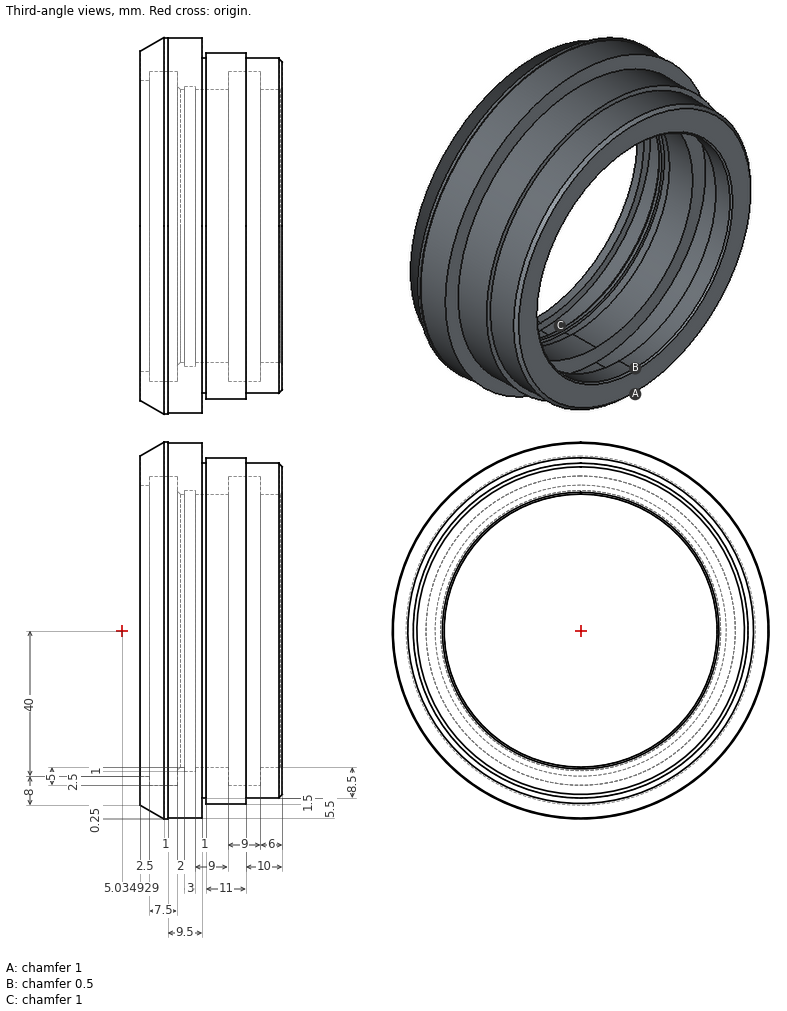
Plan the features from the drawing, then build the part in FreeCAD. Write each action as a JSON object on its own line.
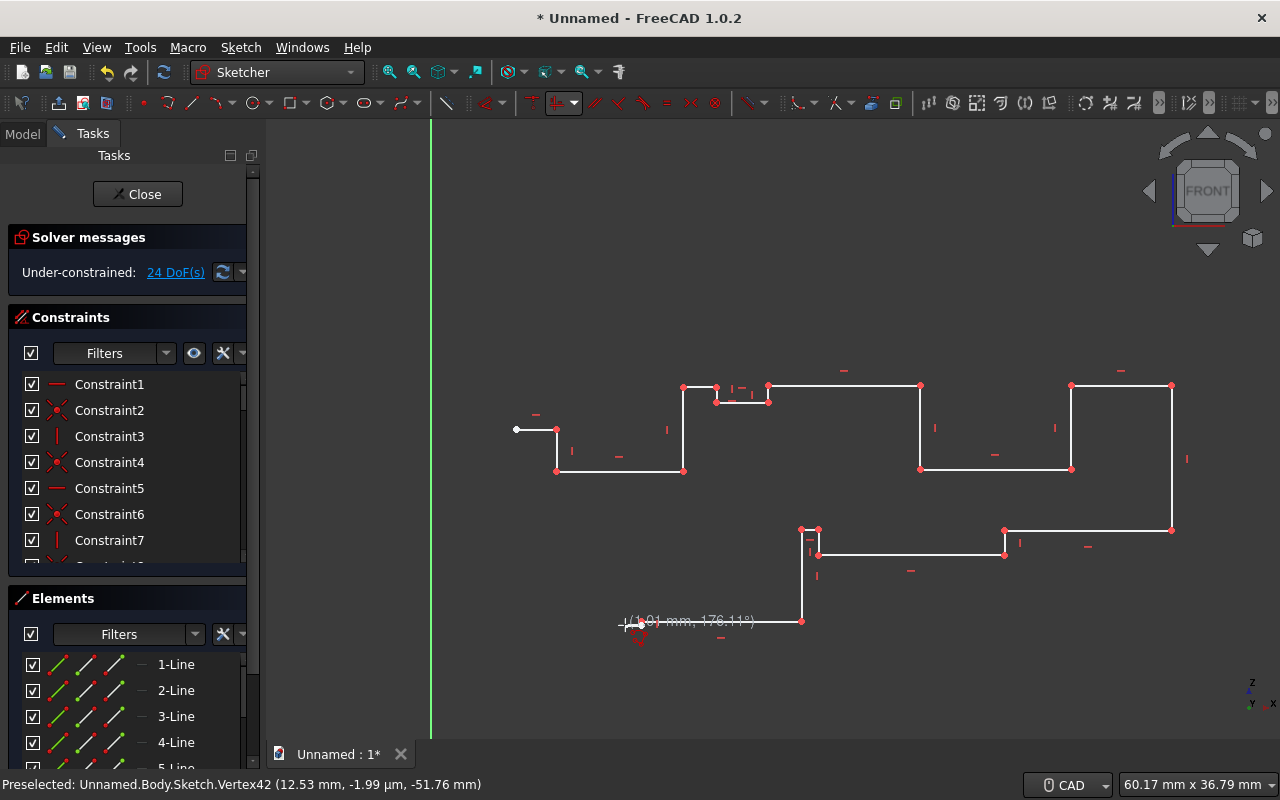
{"action": "left_click", "coordinate": [625, 625]}
{"action": "left_click", "coordinate": [515, 562]}
{"action": "left_click", "coordinate": [516, 430]}
{"action": "key", "text": "Escape"}
{"action": "key", "text": "Escape"}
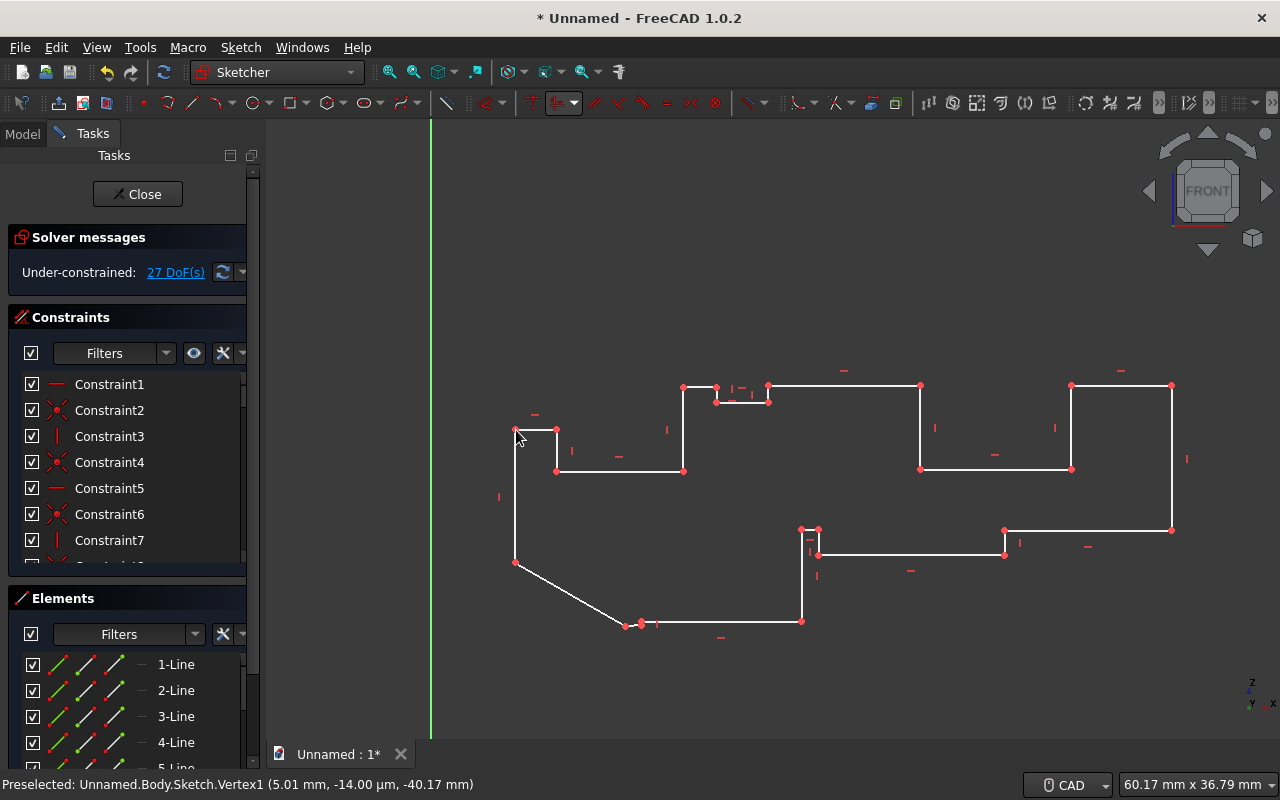
{"action": "scroll", "coordinate": [633, 626], "scroll_direction": "up", "scroll_amount": 3}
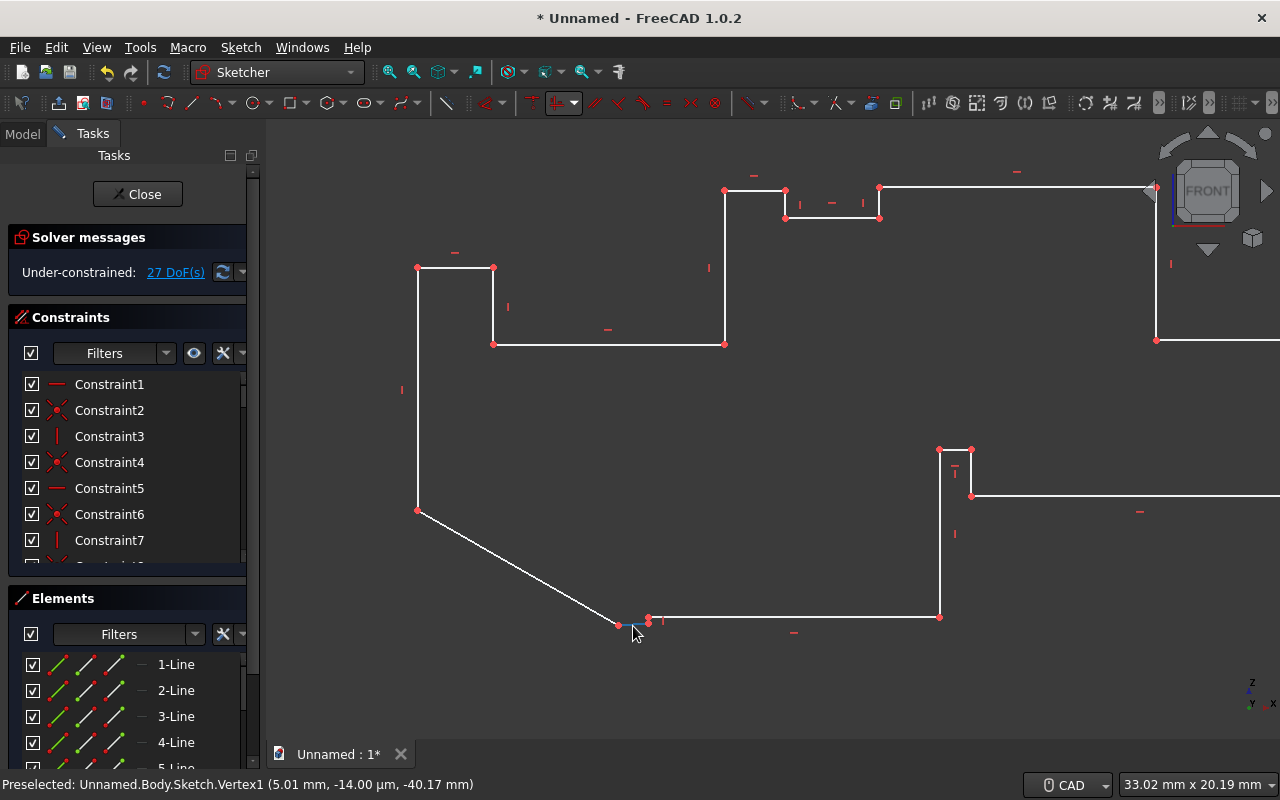
{"action": "left_click", "coordinate": [633, 624]}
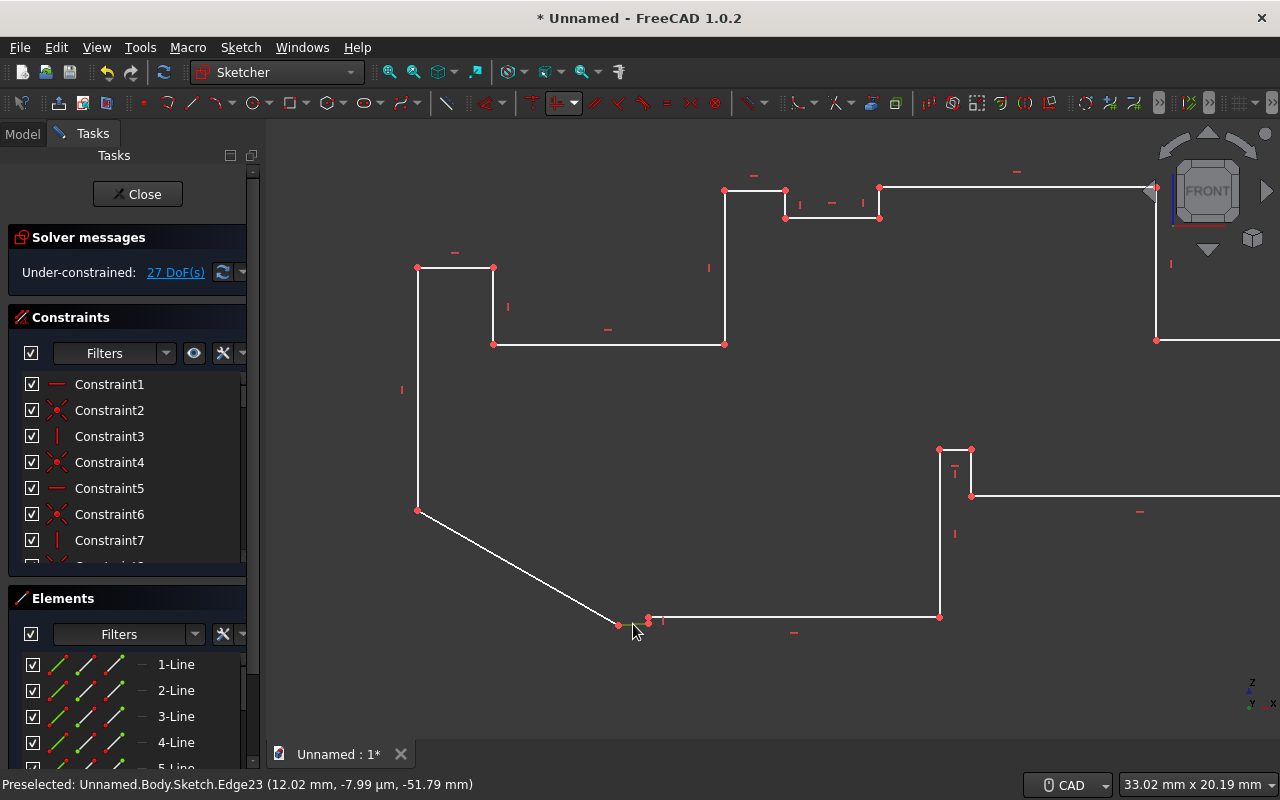
{"action": "key", "text": "h"}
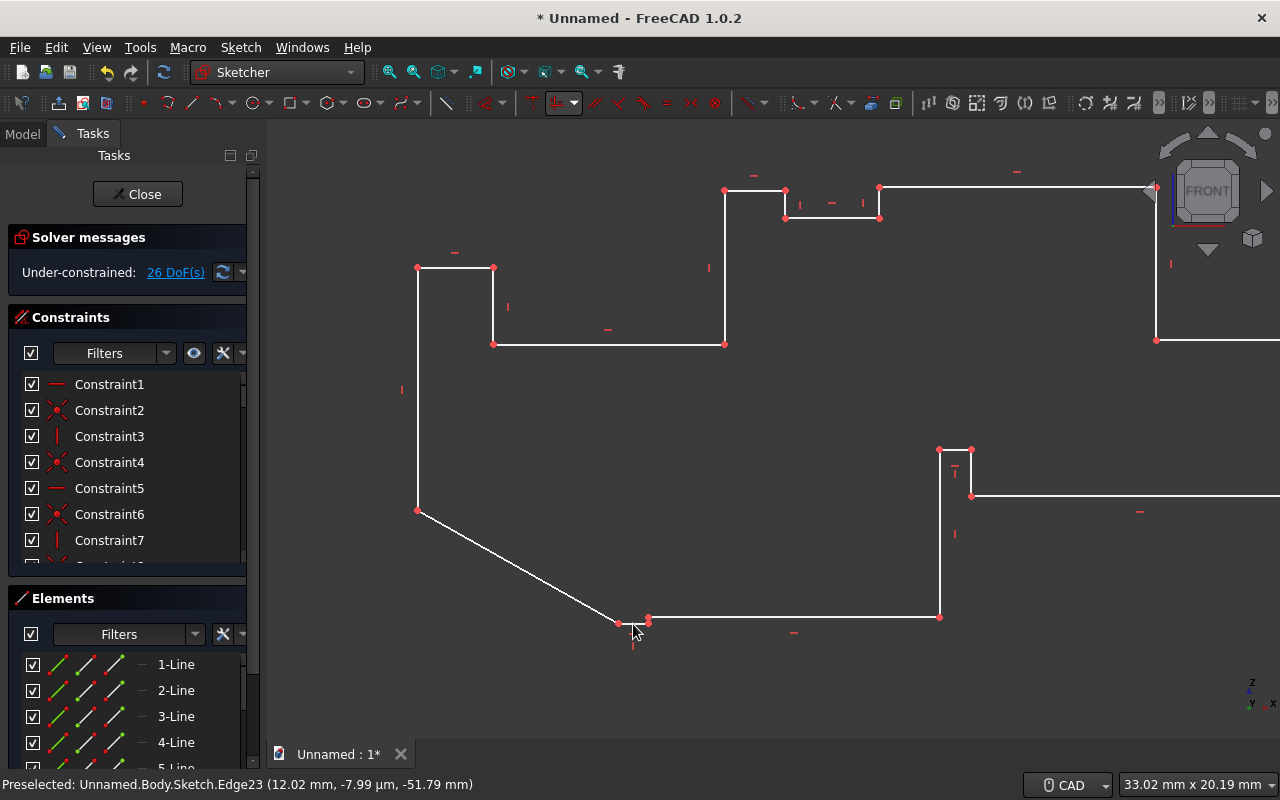
{"action": "key", "text": "d"}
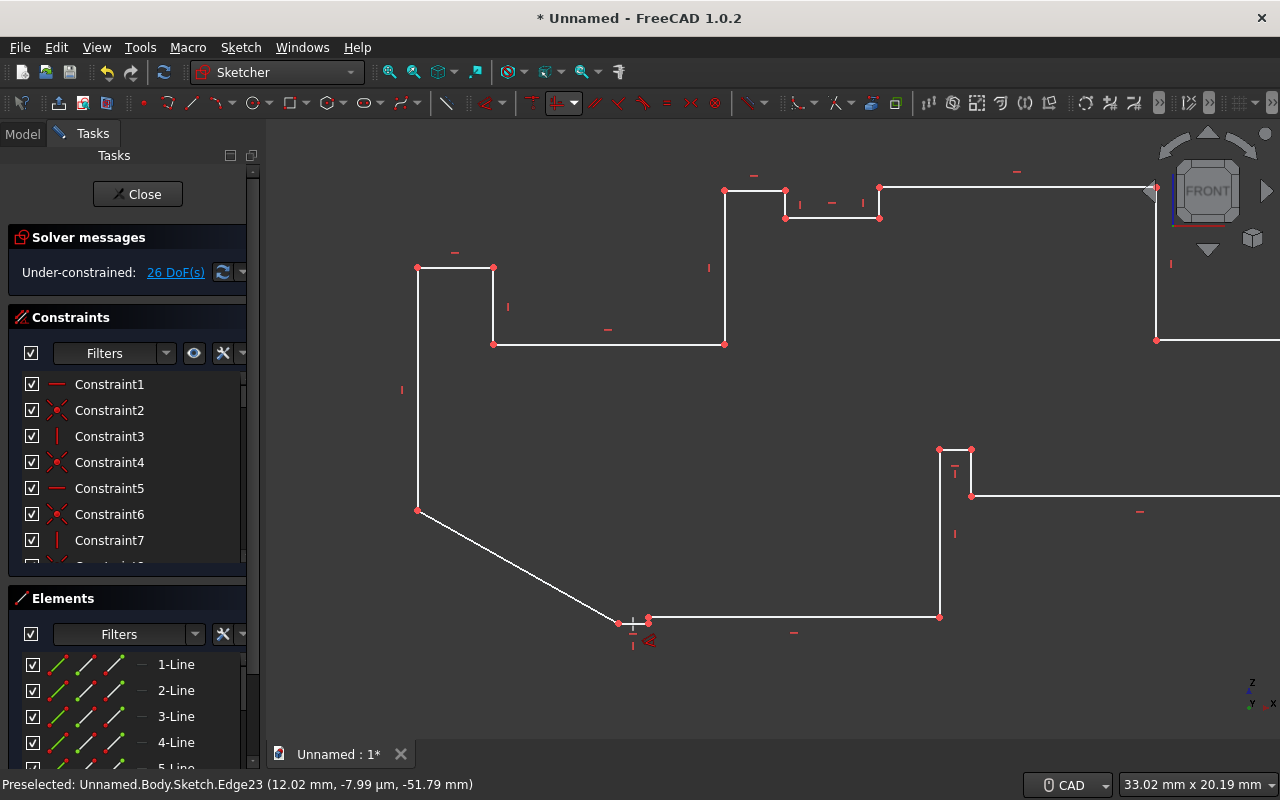
{"action": "scroll", "coordinate": [627, 626], "scroll_direction": "down", "scroll_amount": 7}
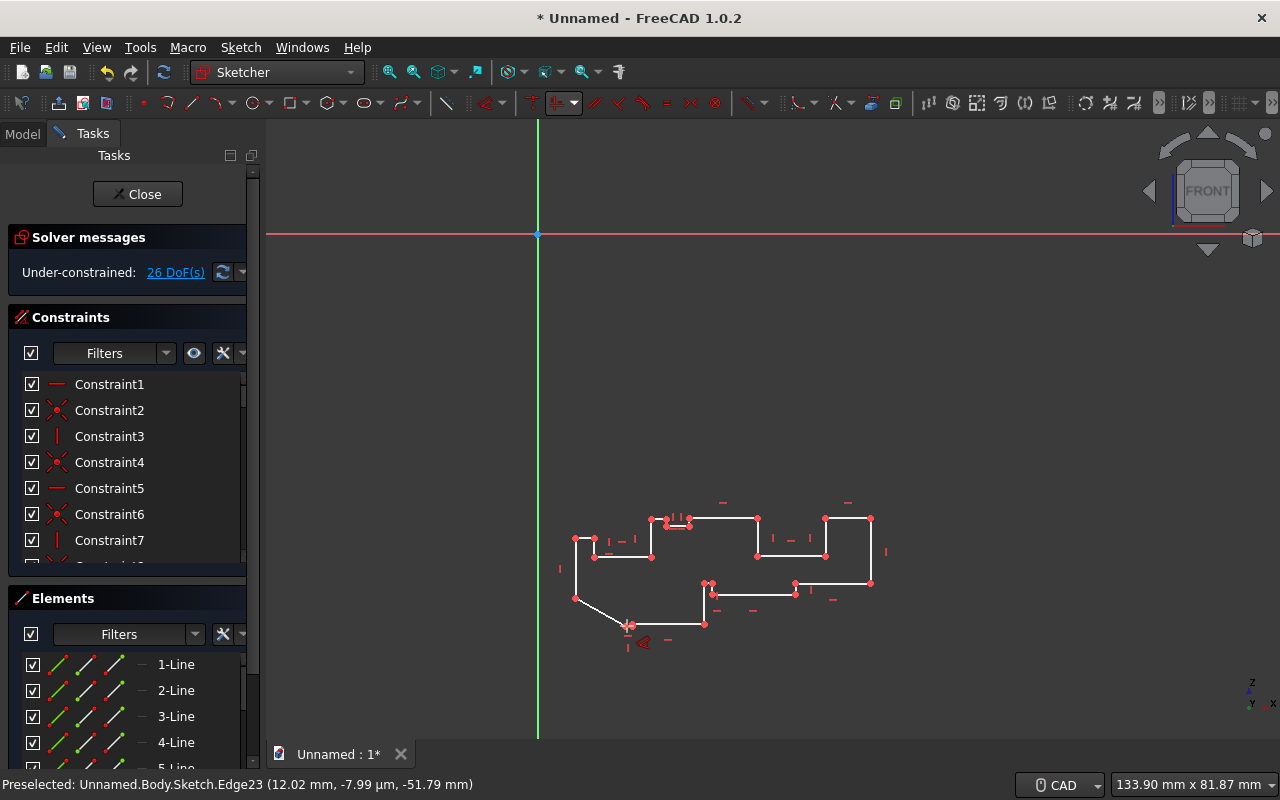
{"action": "left_click", "coordinate": [651, 546]}
{"action": "left_click", "coordinate": [617, 538]}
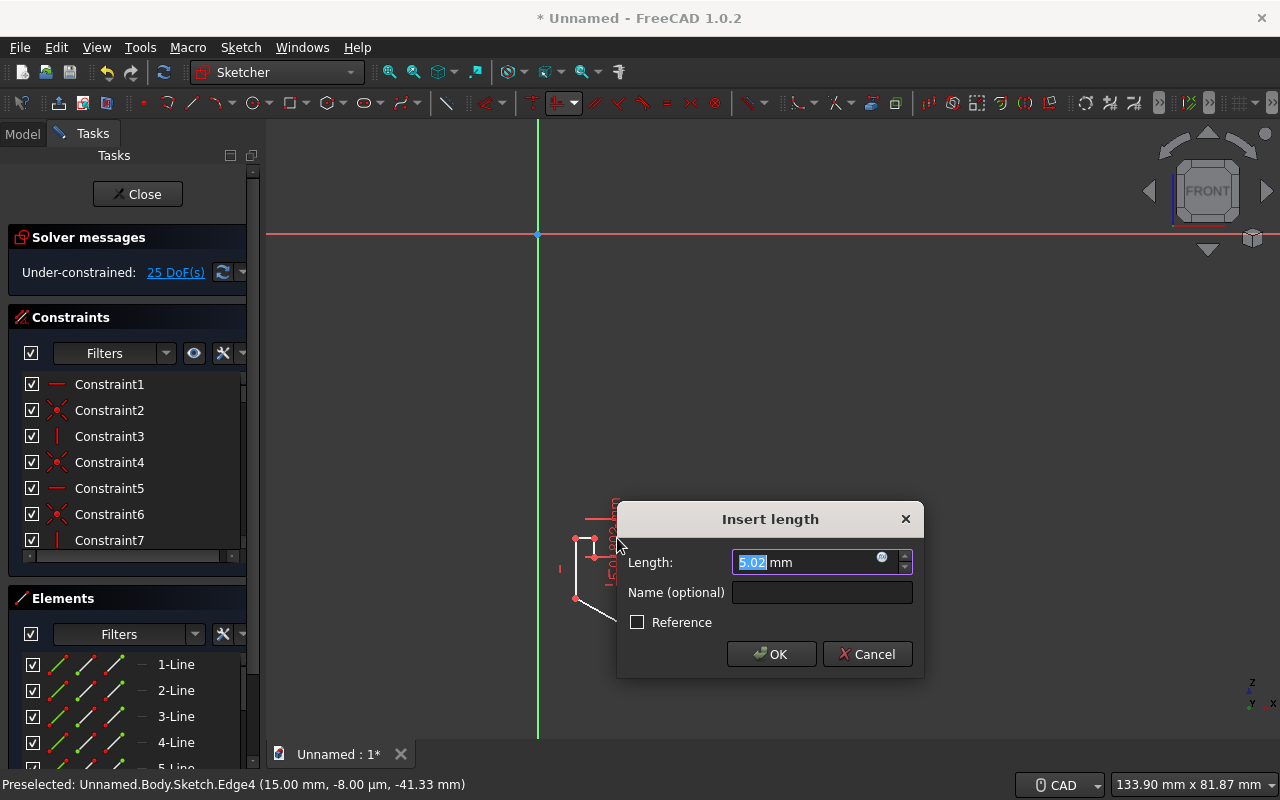
{"action": "type", "text": "5"}
{"action": "key", "text": "Return"}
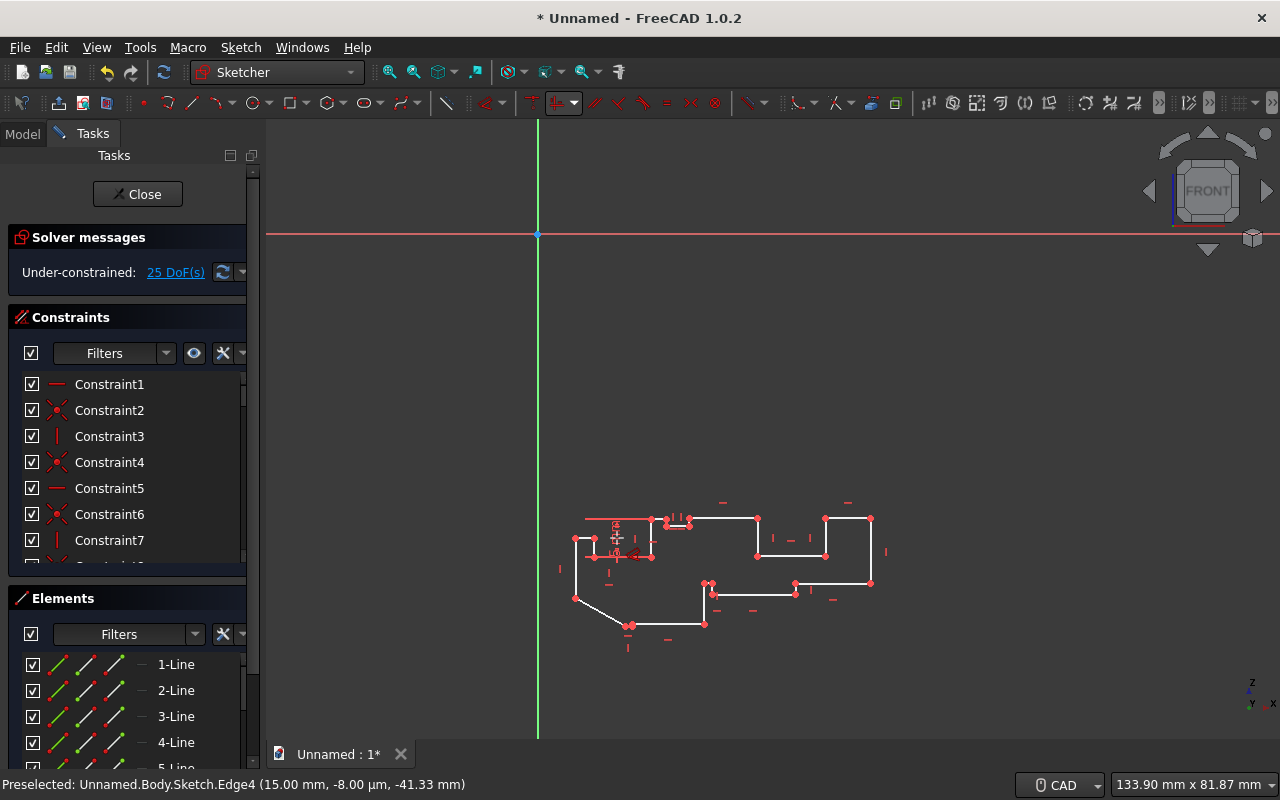
{"action": "scroll", "coordinate": [659, 519], "scroll_direction": "up", "scroll_amount": 5}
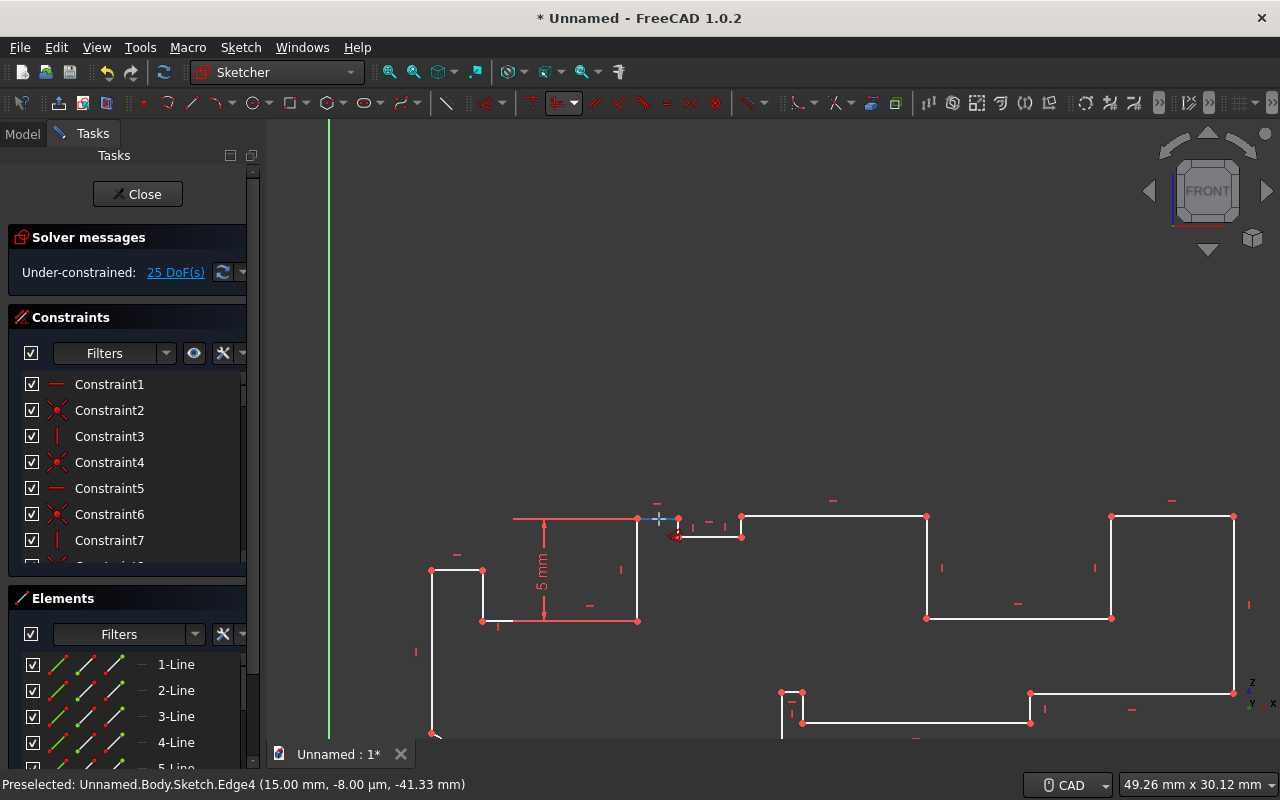
{"action": "left_click", "coordinate": [658, 519]}
{"action": "left_click", "coordinate": [658, 553]}